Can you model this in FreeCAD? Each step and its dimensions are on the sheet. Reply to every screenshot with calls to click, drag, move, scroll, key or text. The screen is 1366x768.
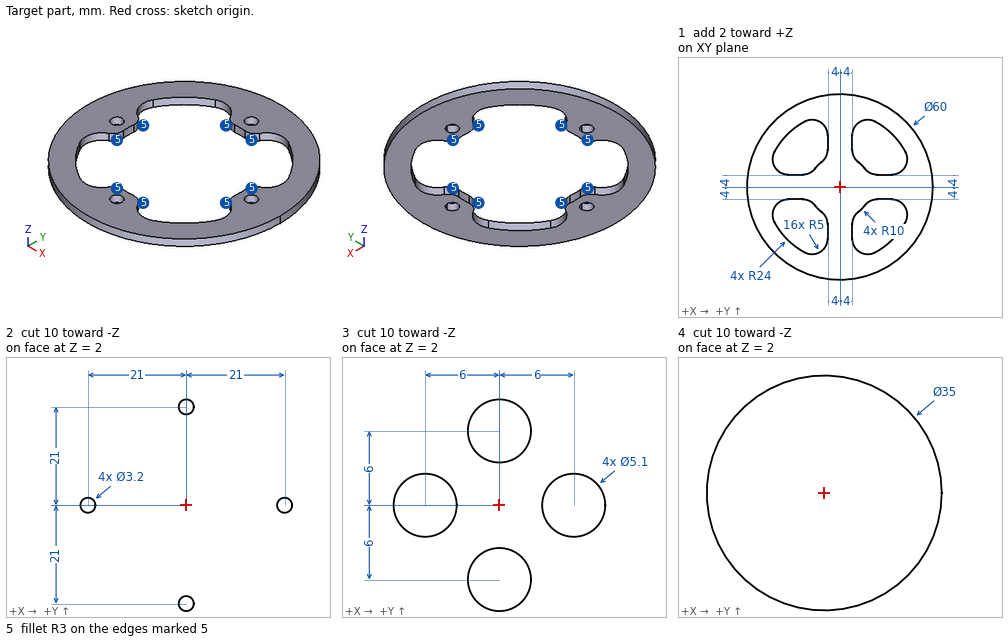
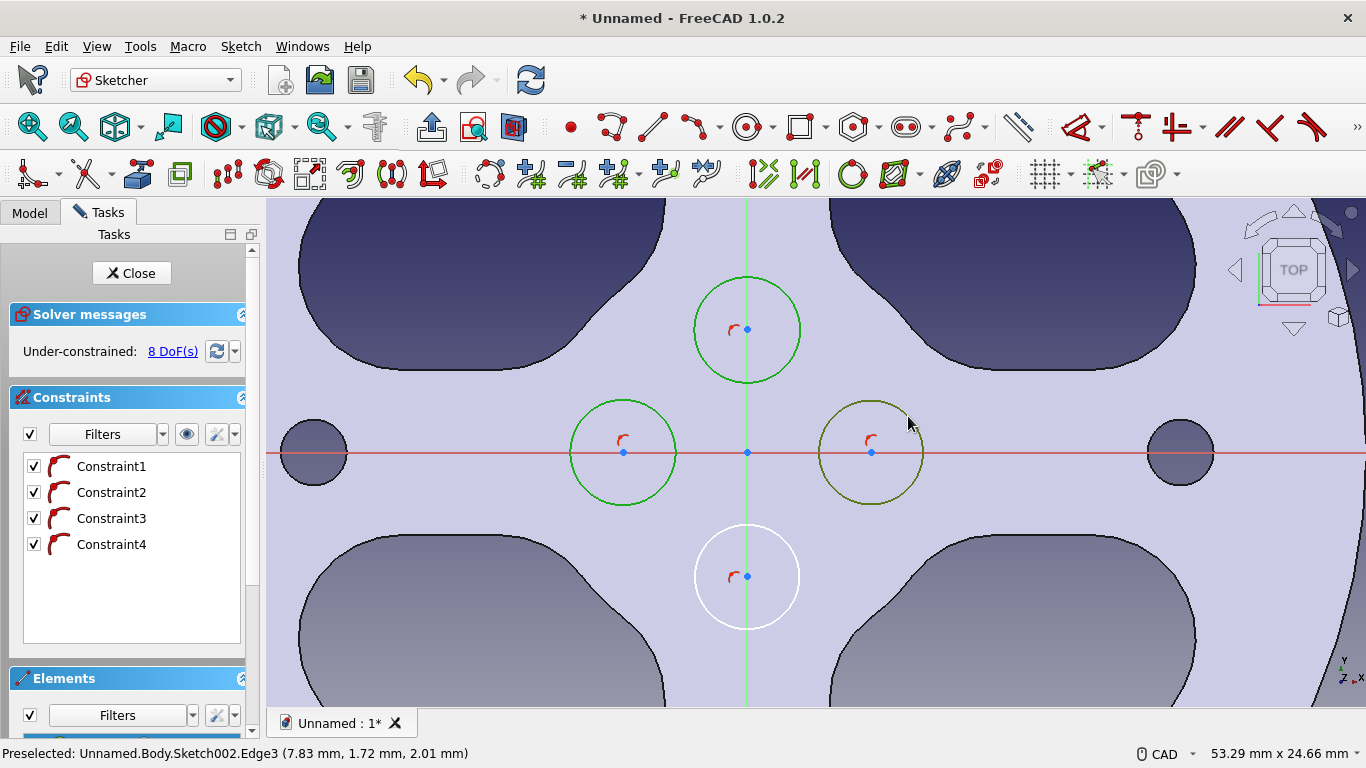
click(784, 540)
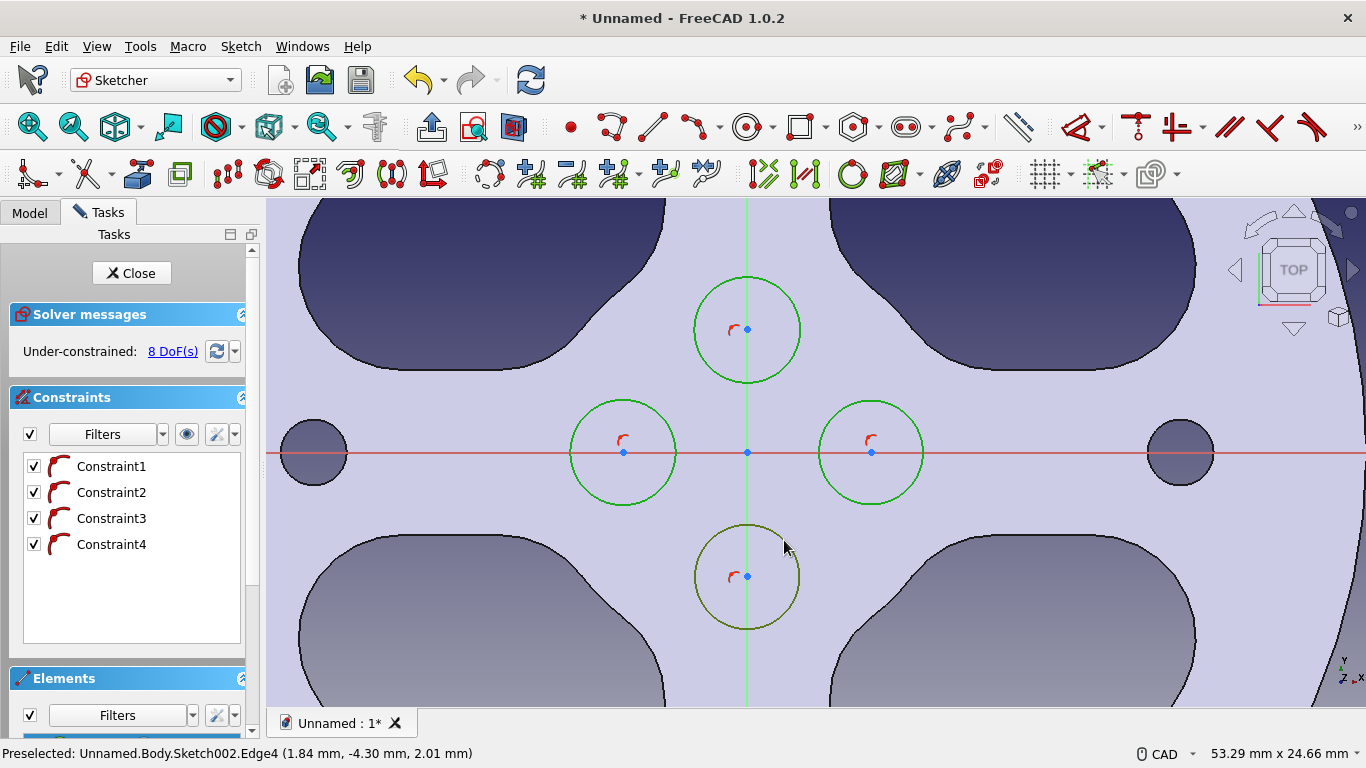
key(e)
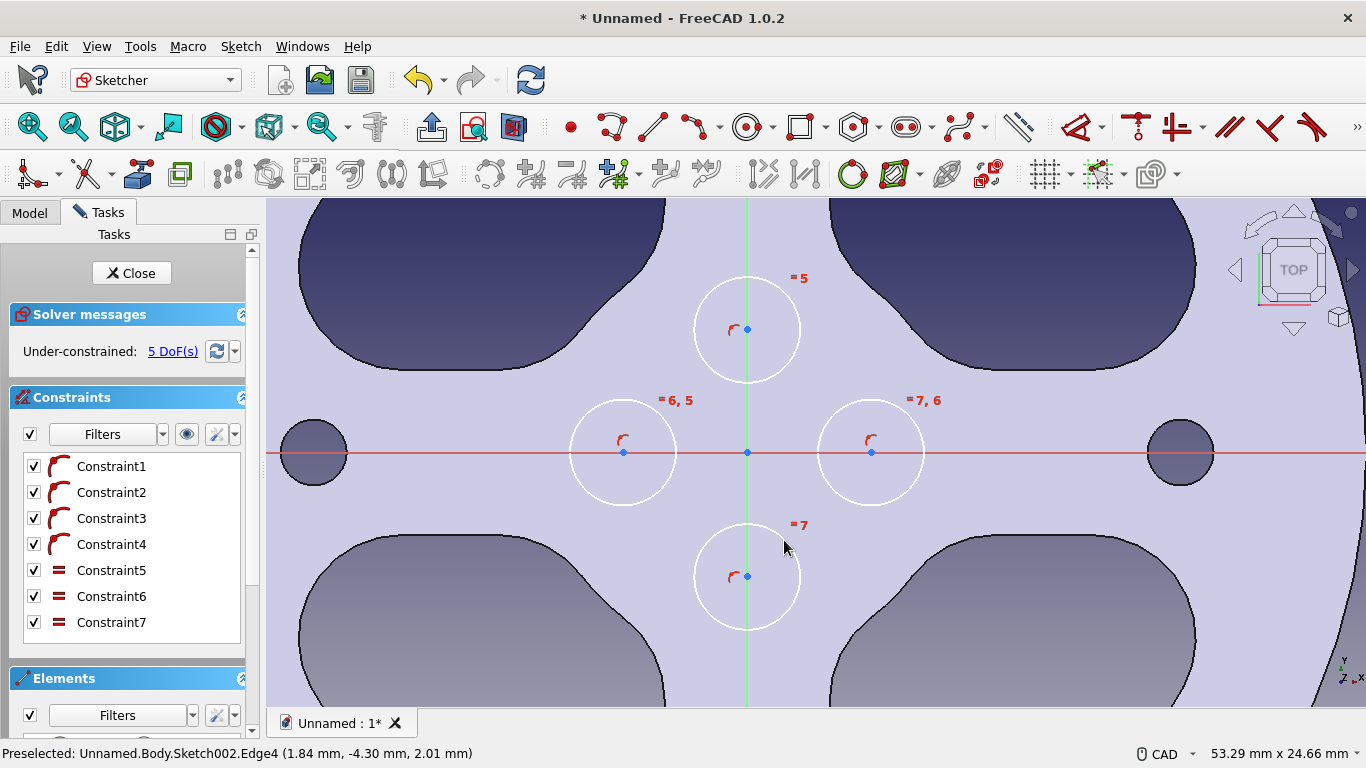
click(1076, 128)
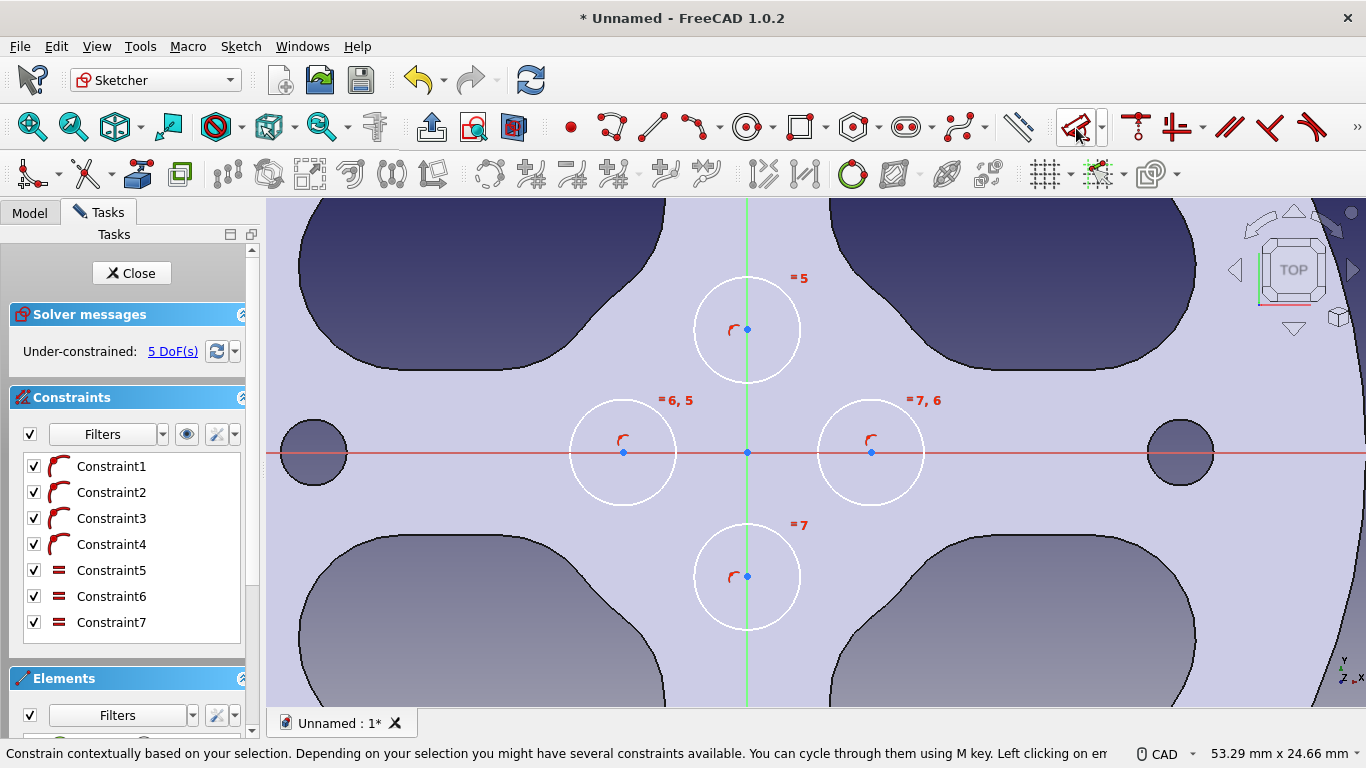
click(784, 292)
click(806, 269)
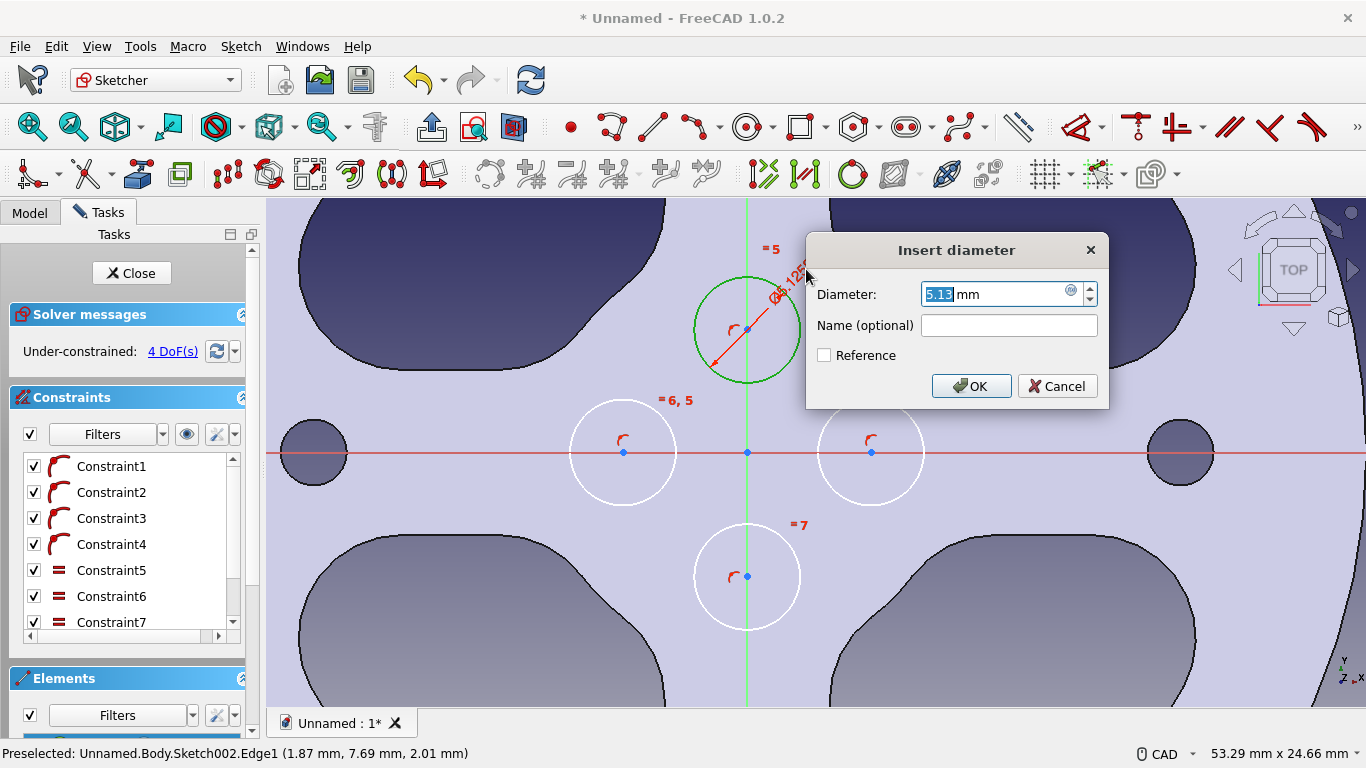
text(5.1)
key(Return)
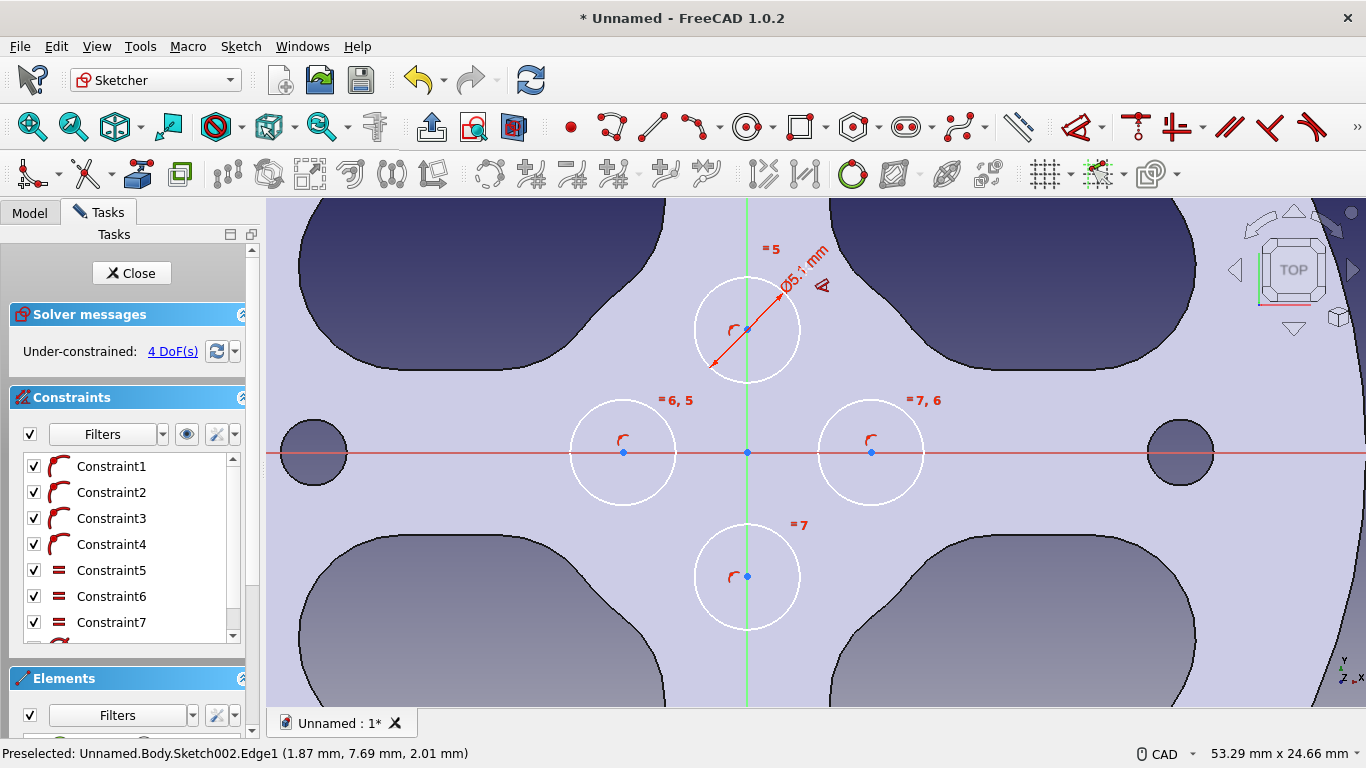
click(747, 330)
click(781, 391)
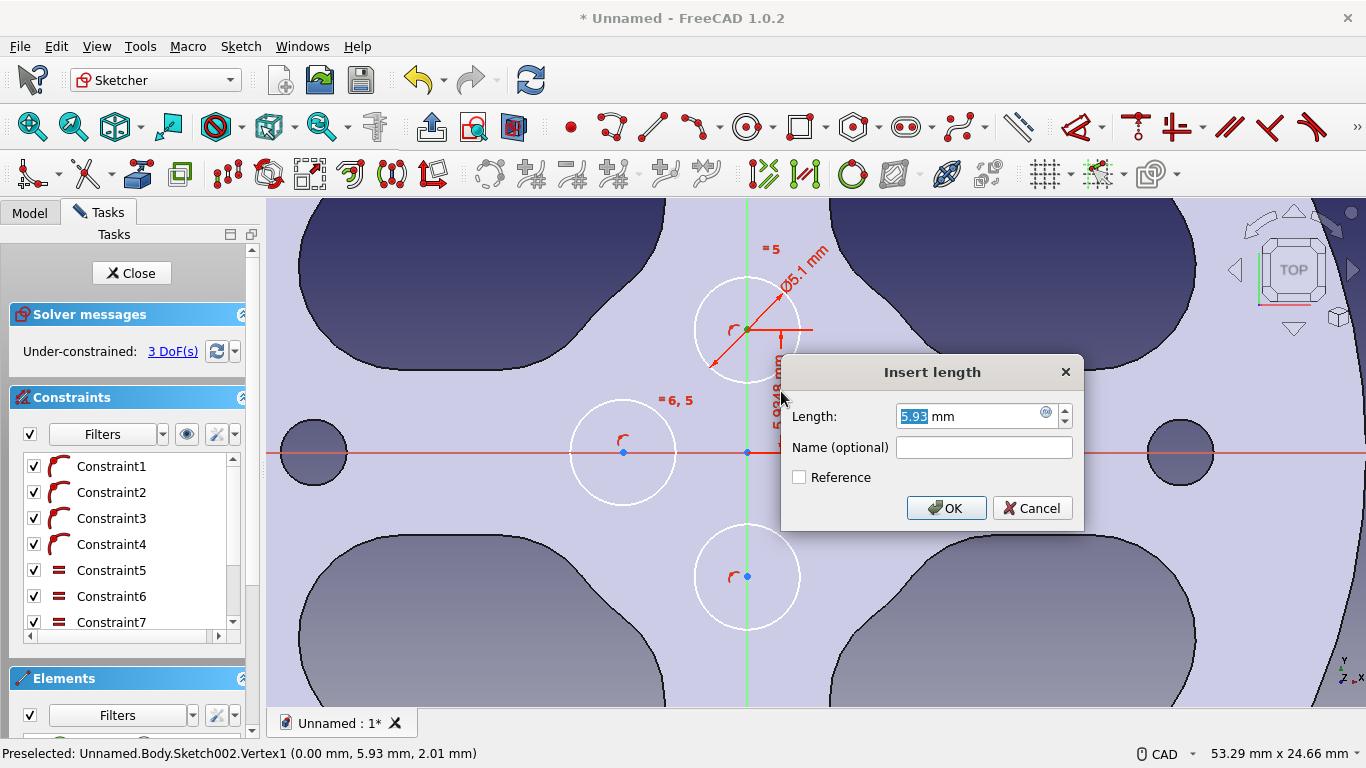
text(6)
key(Return)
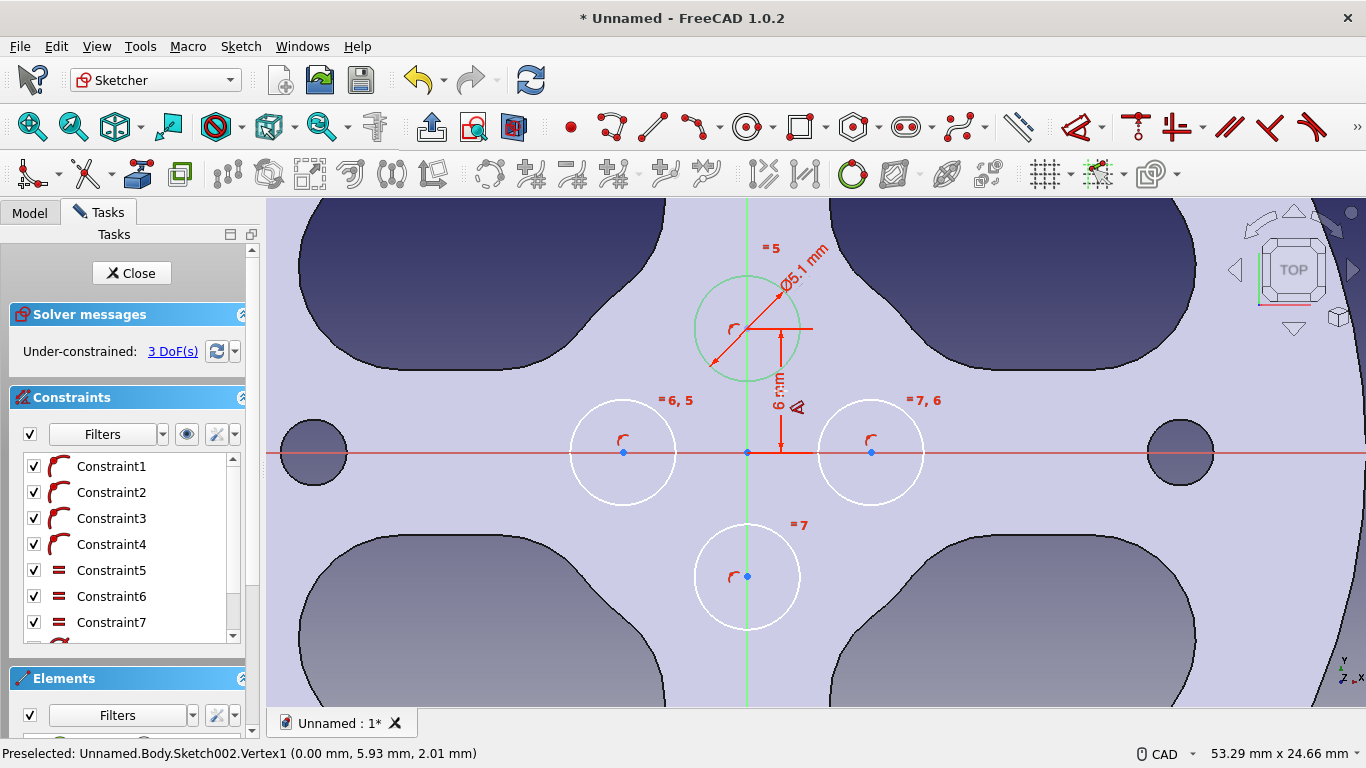
click(623, 452)
click(685, 486)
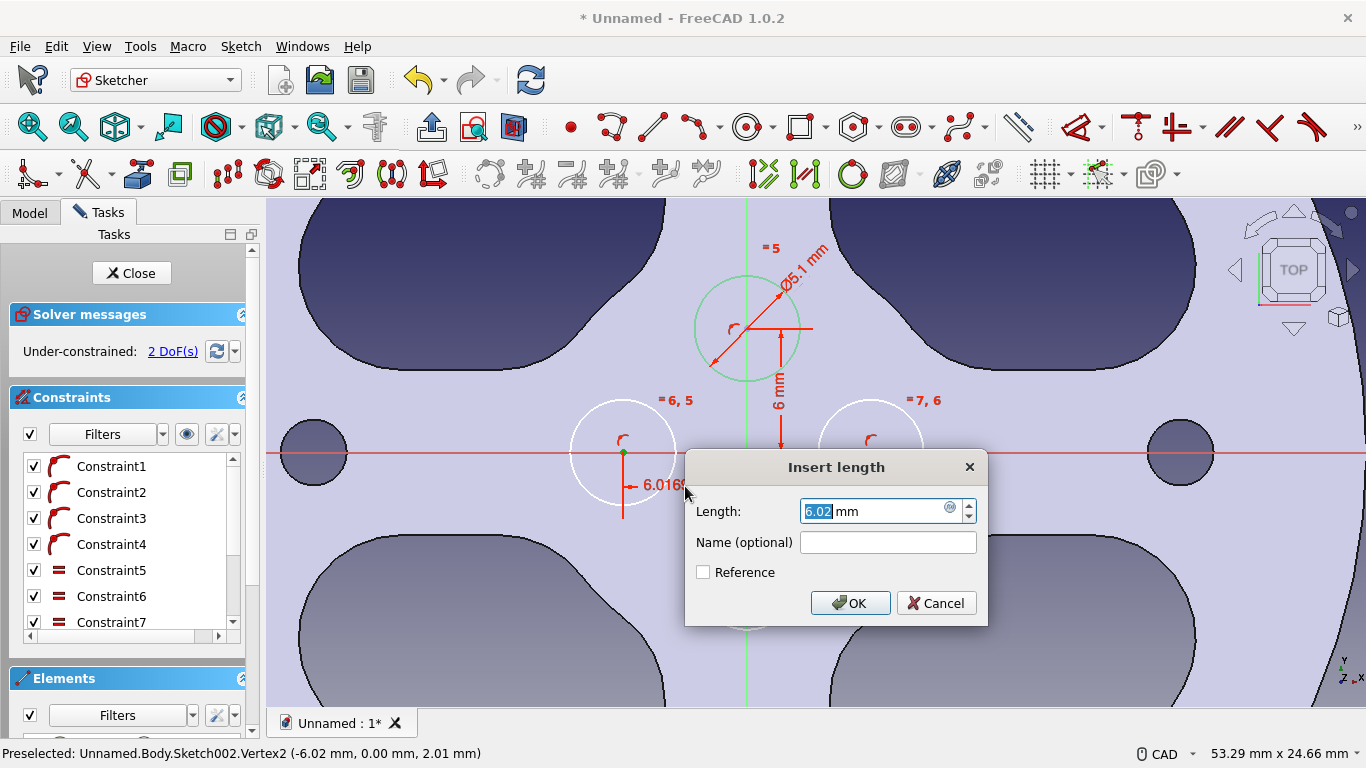
text(6)
key(Return)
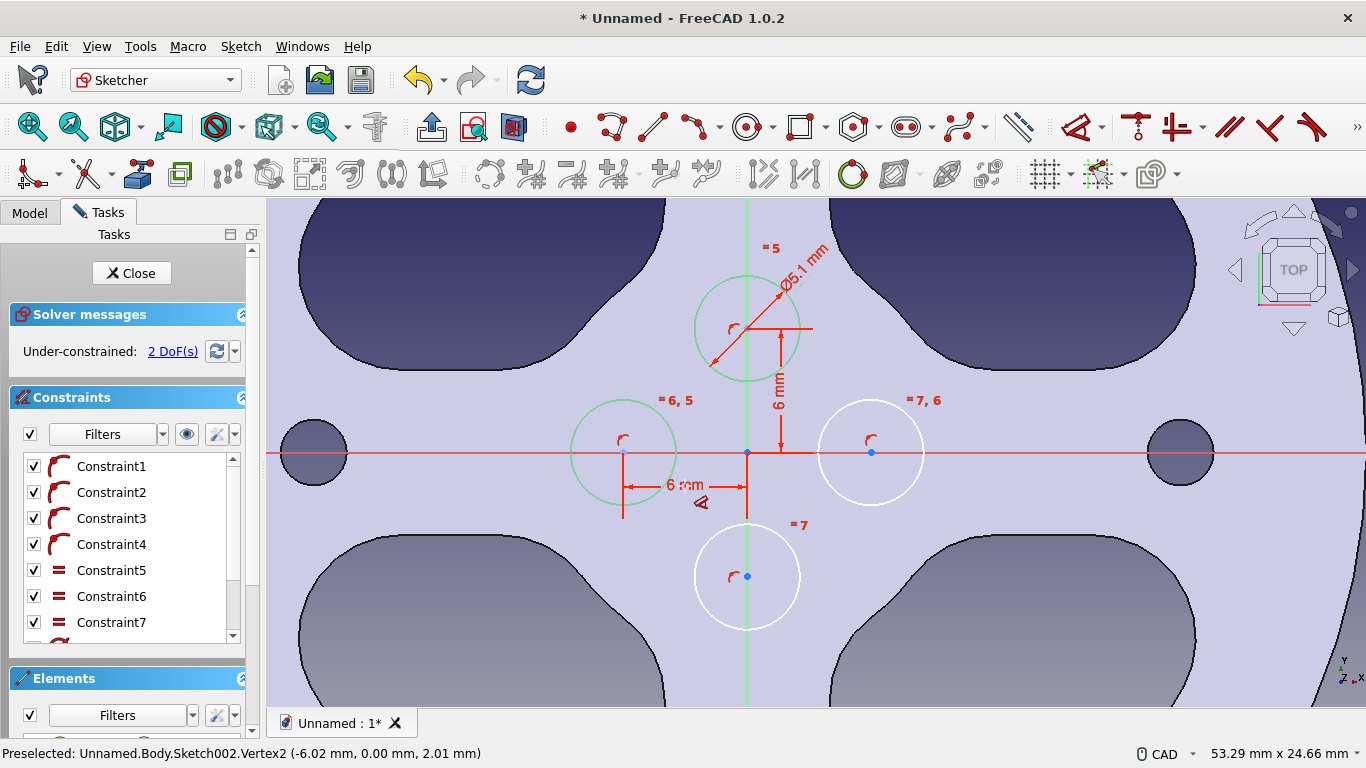
click(871, 452)
click(809, 486)